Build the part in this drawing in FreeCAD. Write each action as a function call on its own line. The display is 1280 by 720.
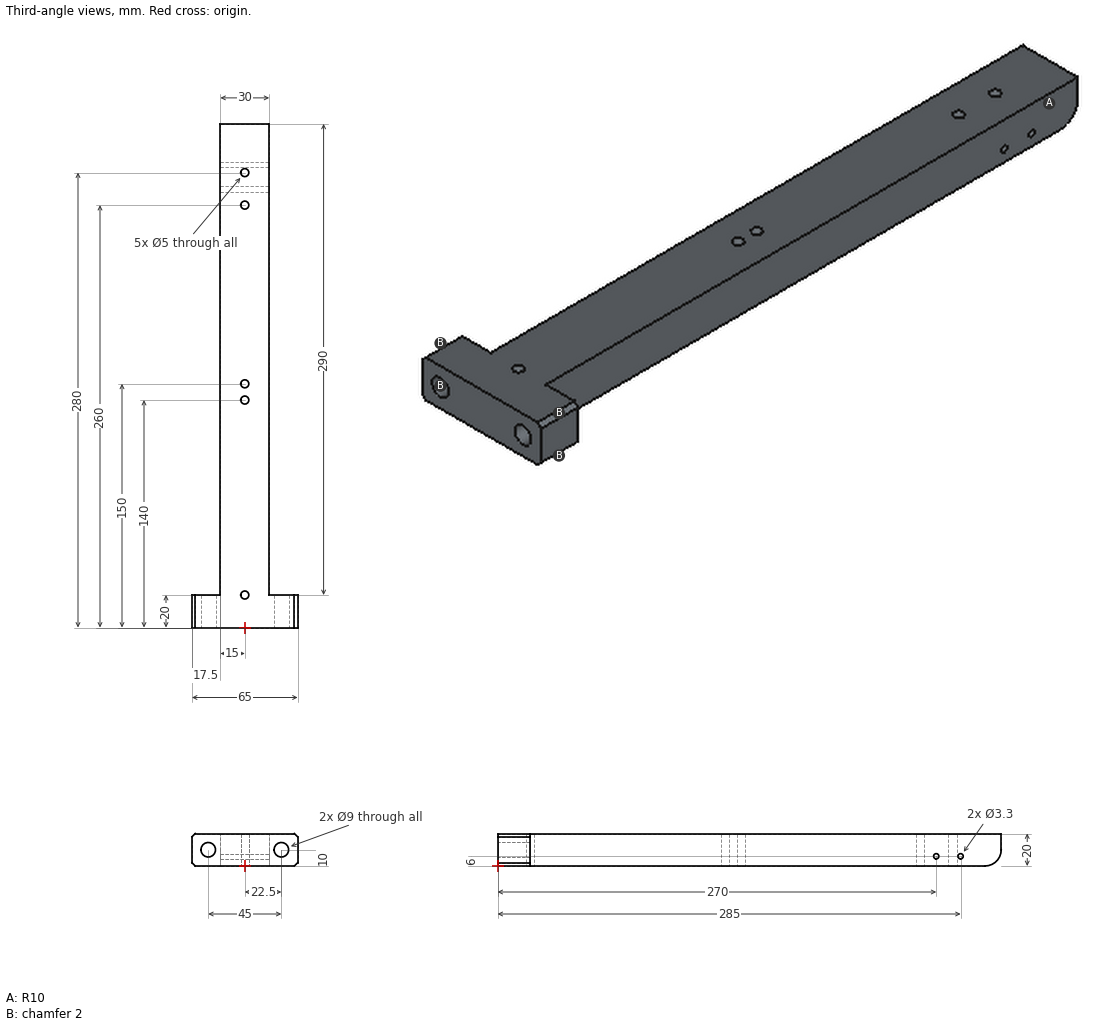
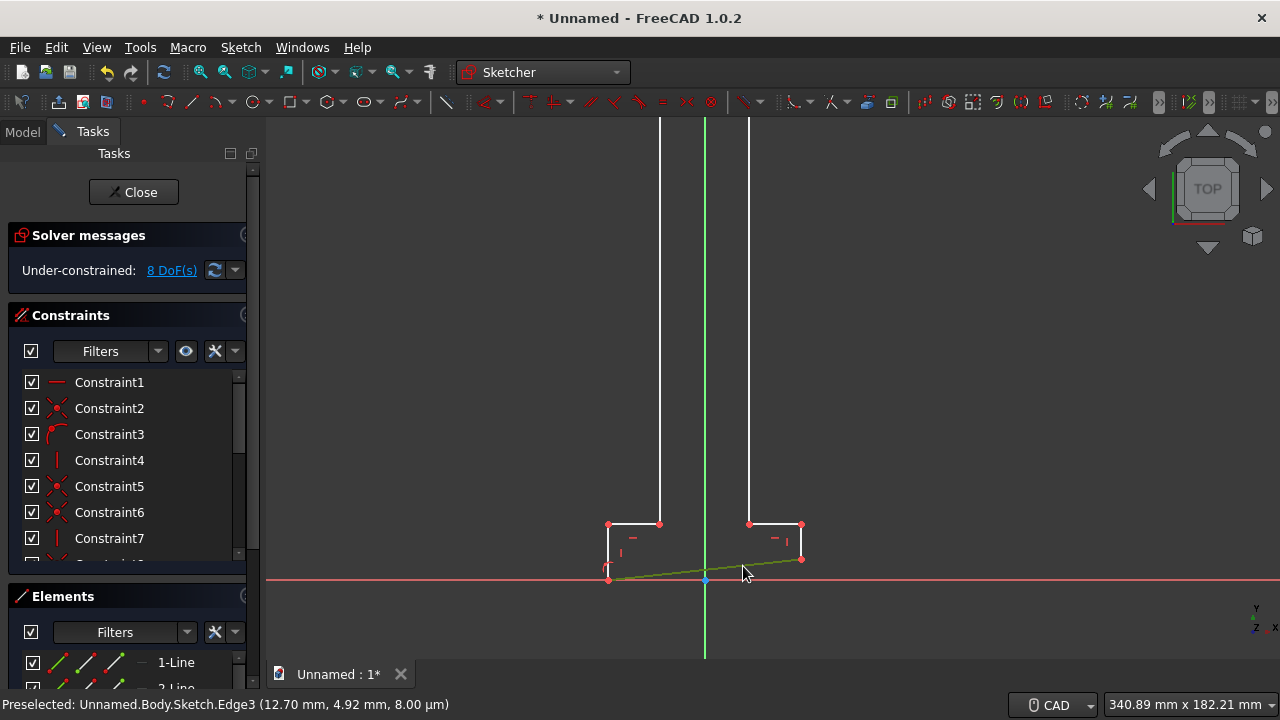
click(572, 102)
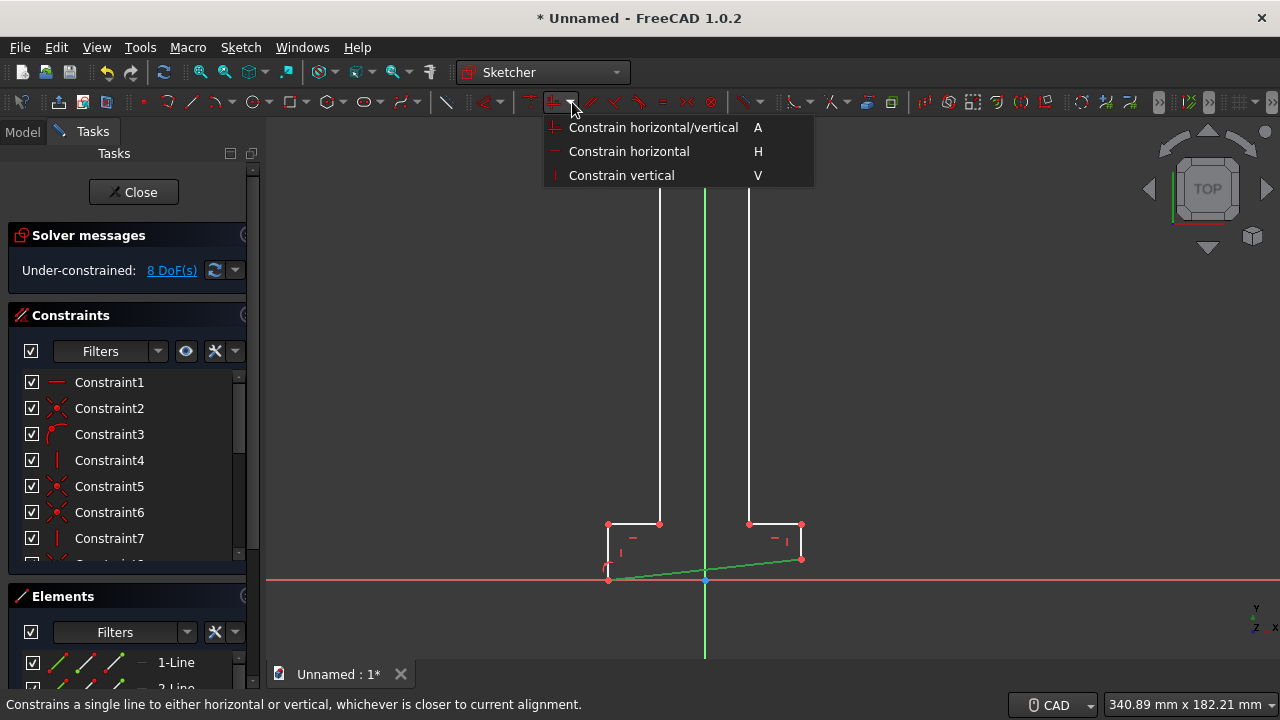
click(679, 151)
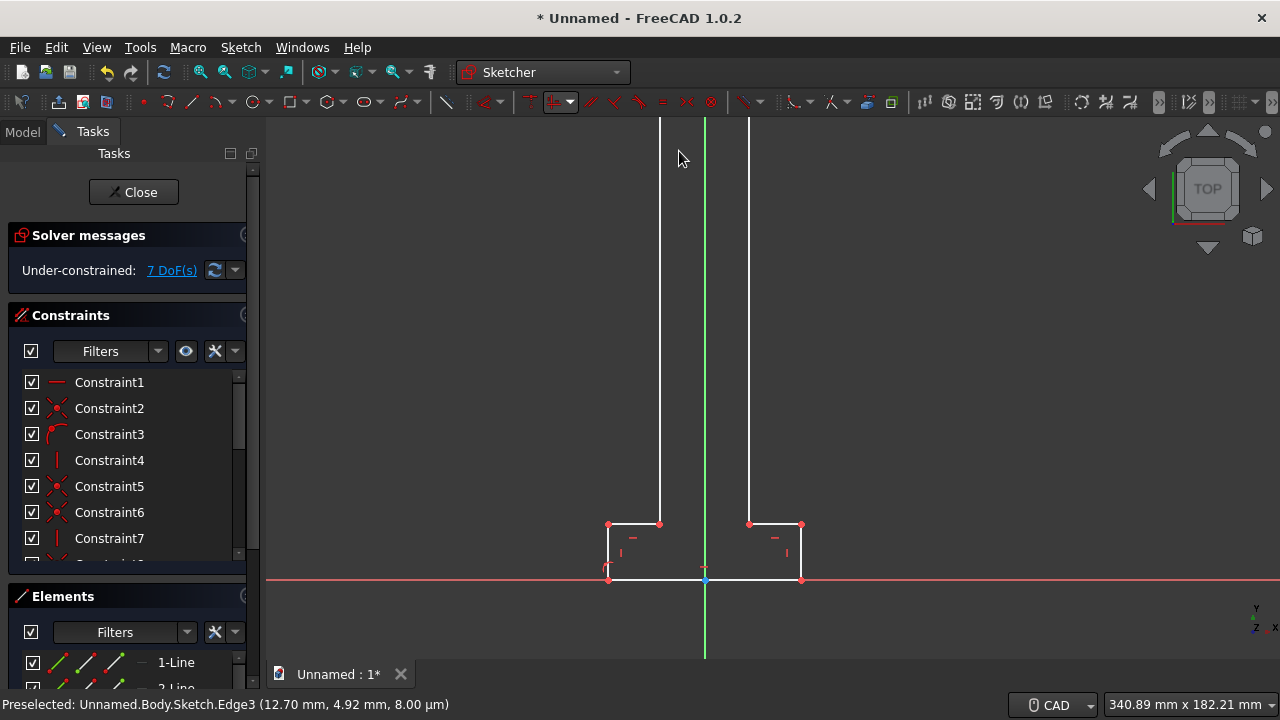
click(484, 102)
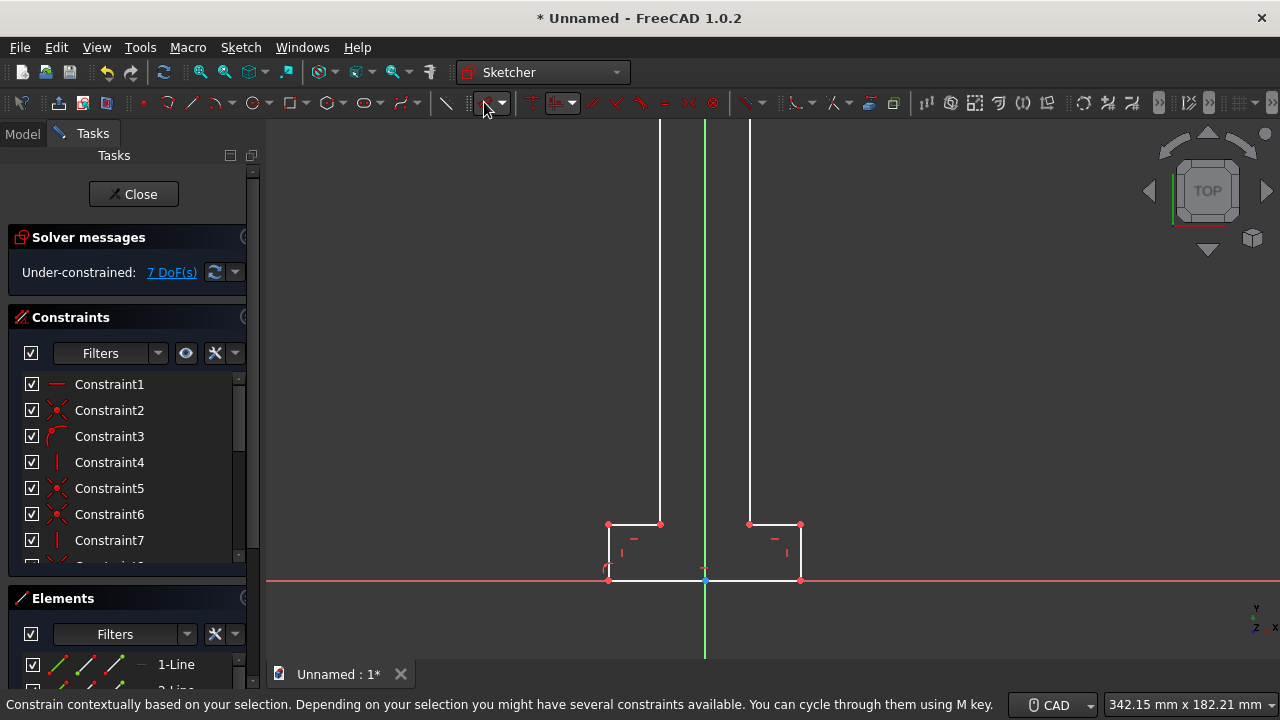
click(609, 541)
click(575, 553)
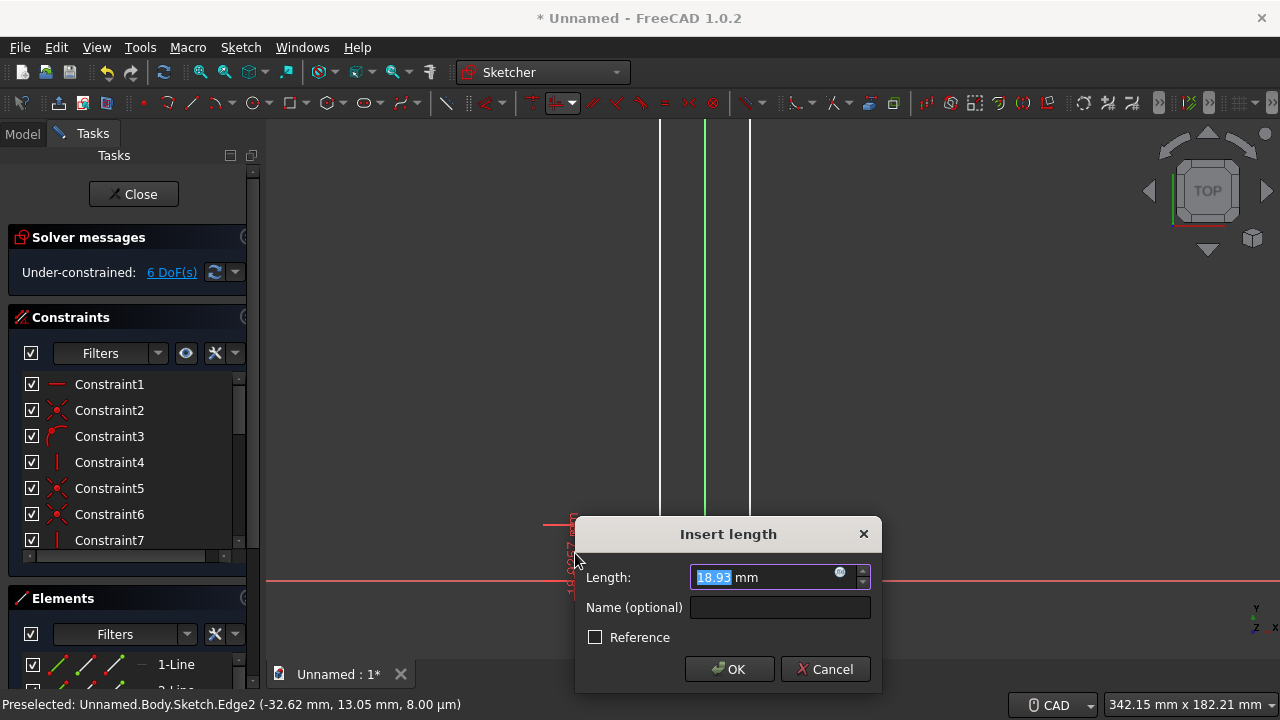
text(20)
key(Return)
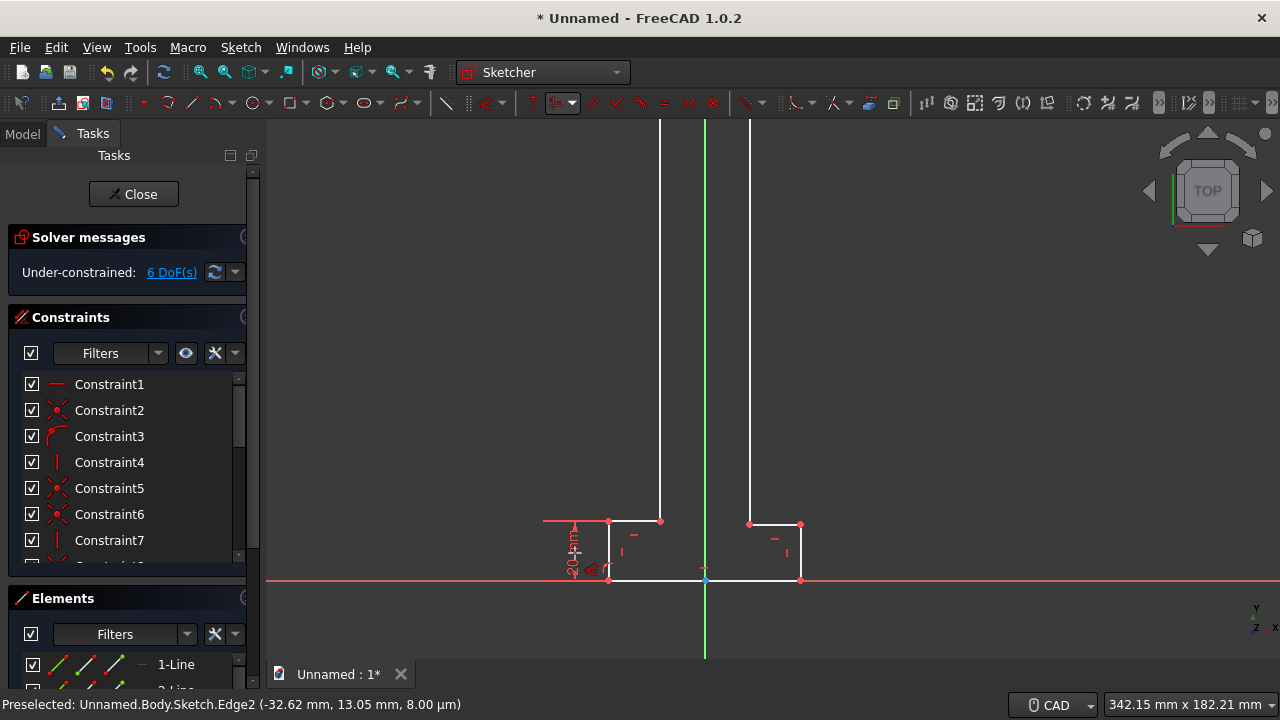
click(666, 581)
click(661, 615)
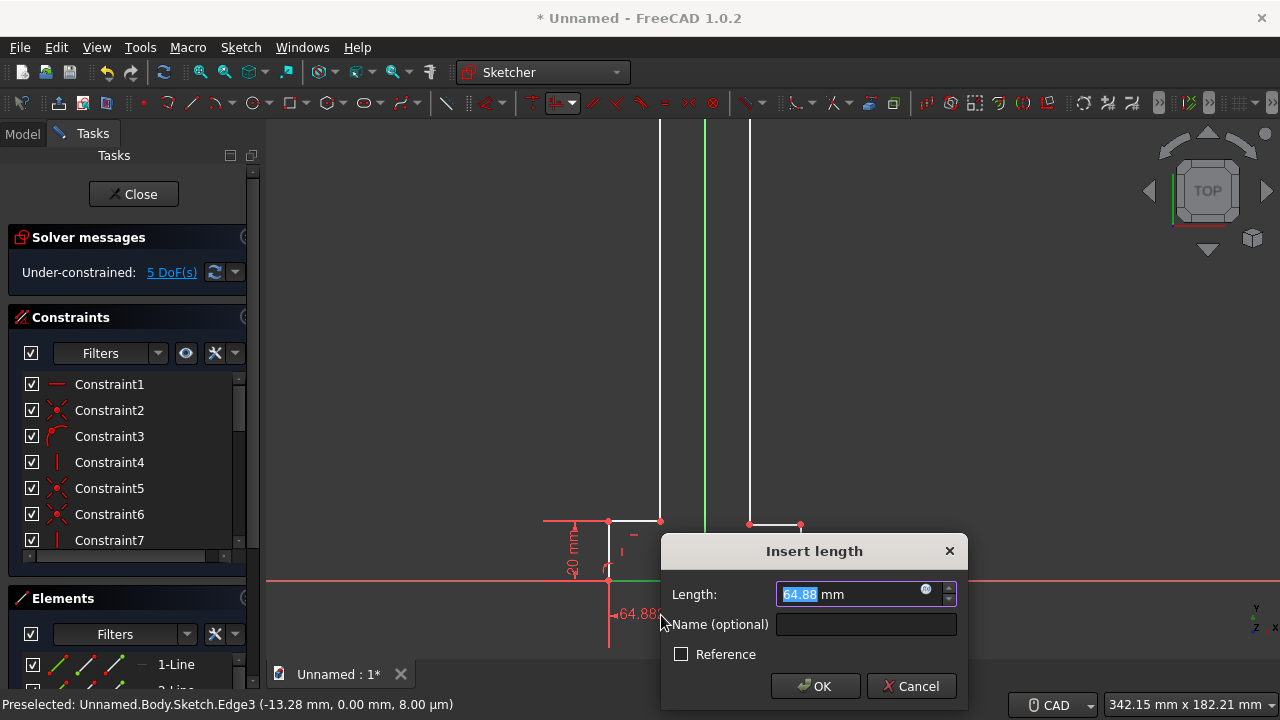
text(65)
key(Return)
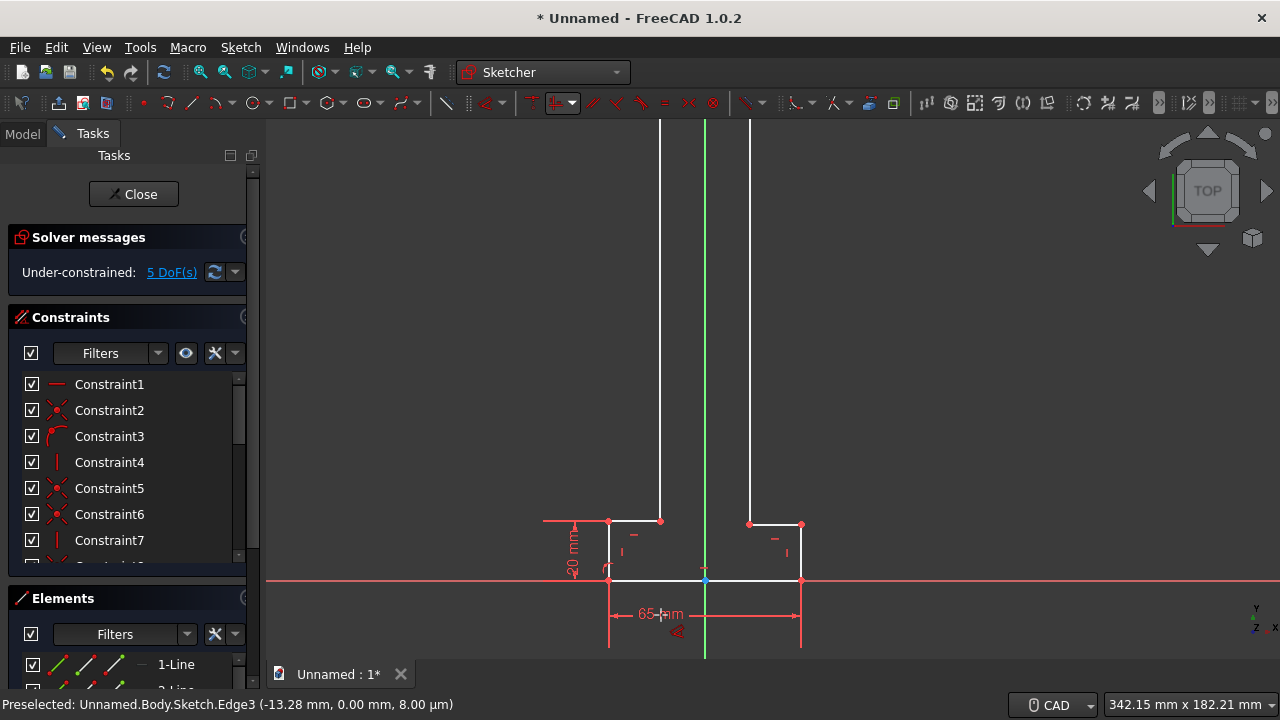
click(801, 564)
click(835, 553)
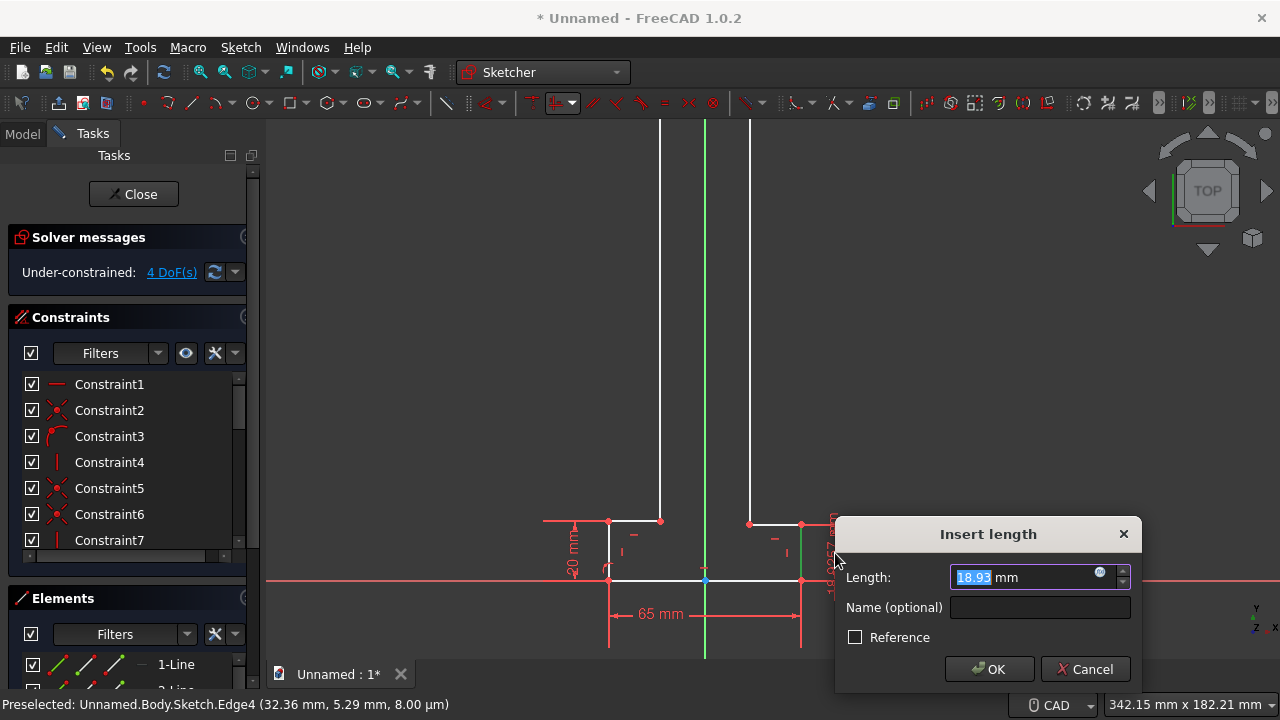
text(20)
key(Return)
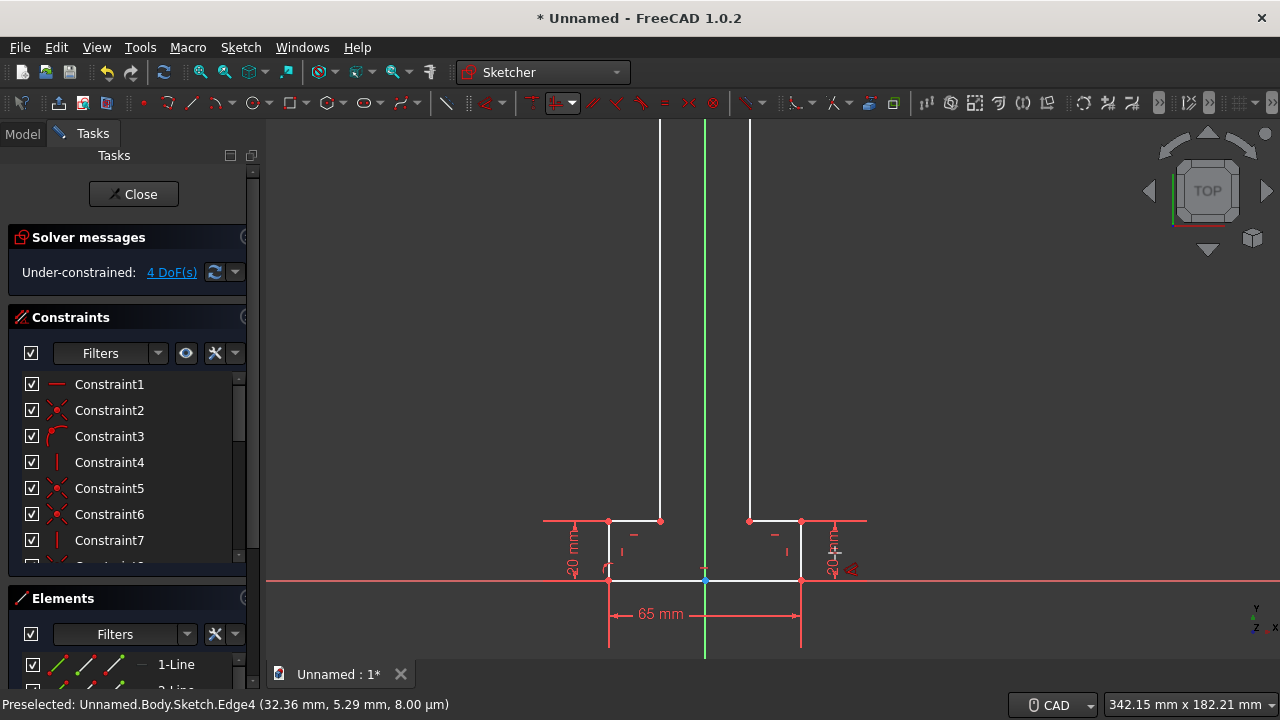
scroll(704, 545, down, 5)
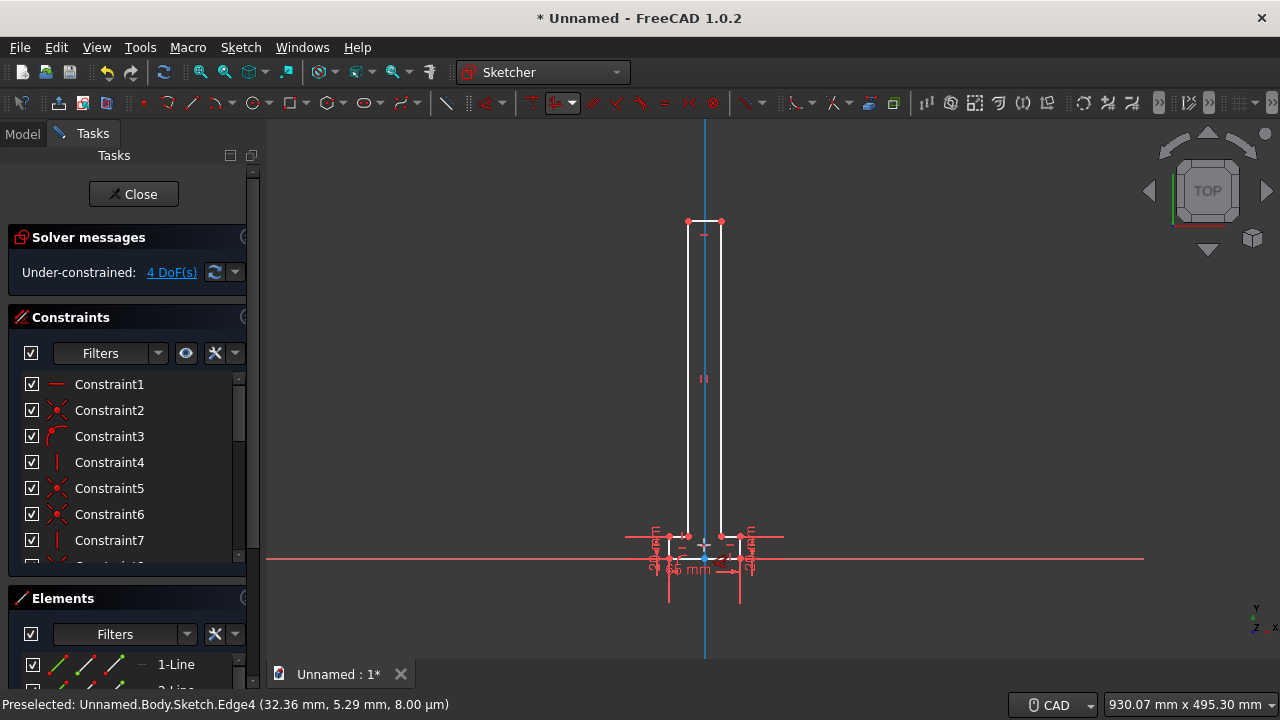
scroll(711, 221, up, 4)